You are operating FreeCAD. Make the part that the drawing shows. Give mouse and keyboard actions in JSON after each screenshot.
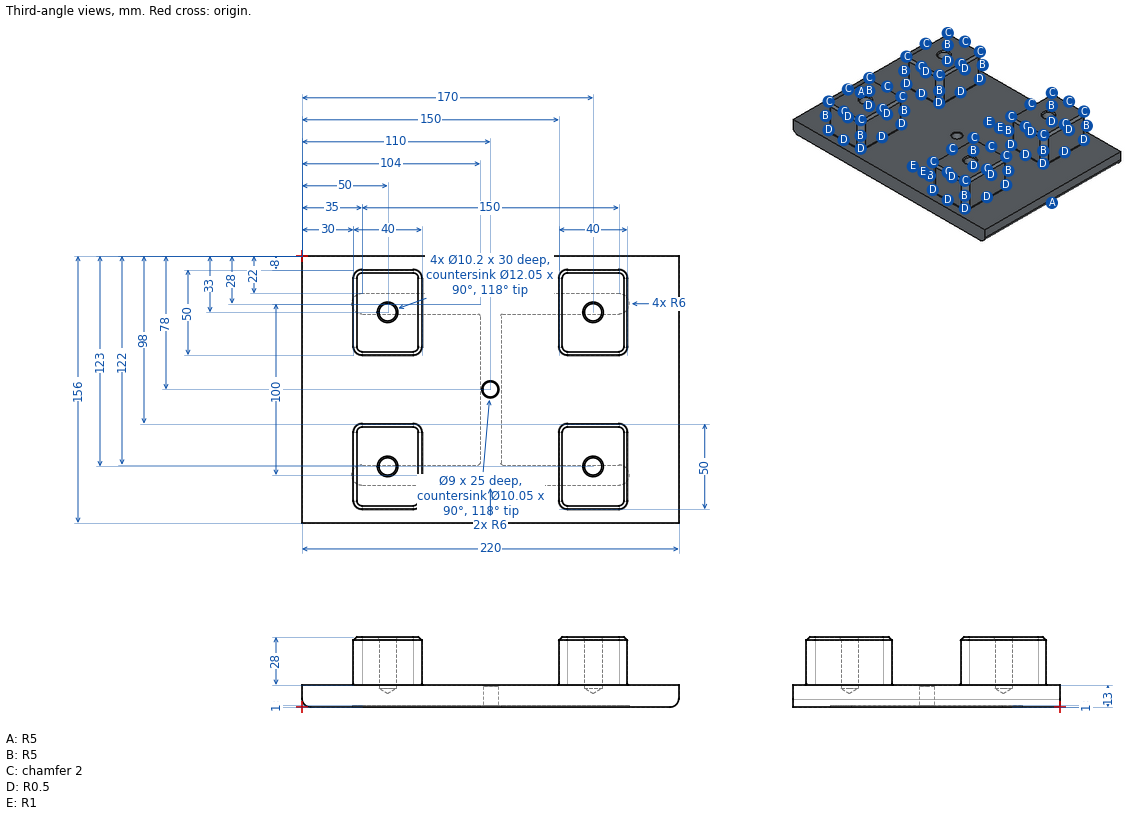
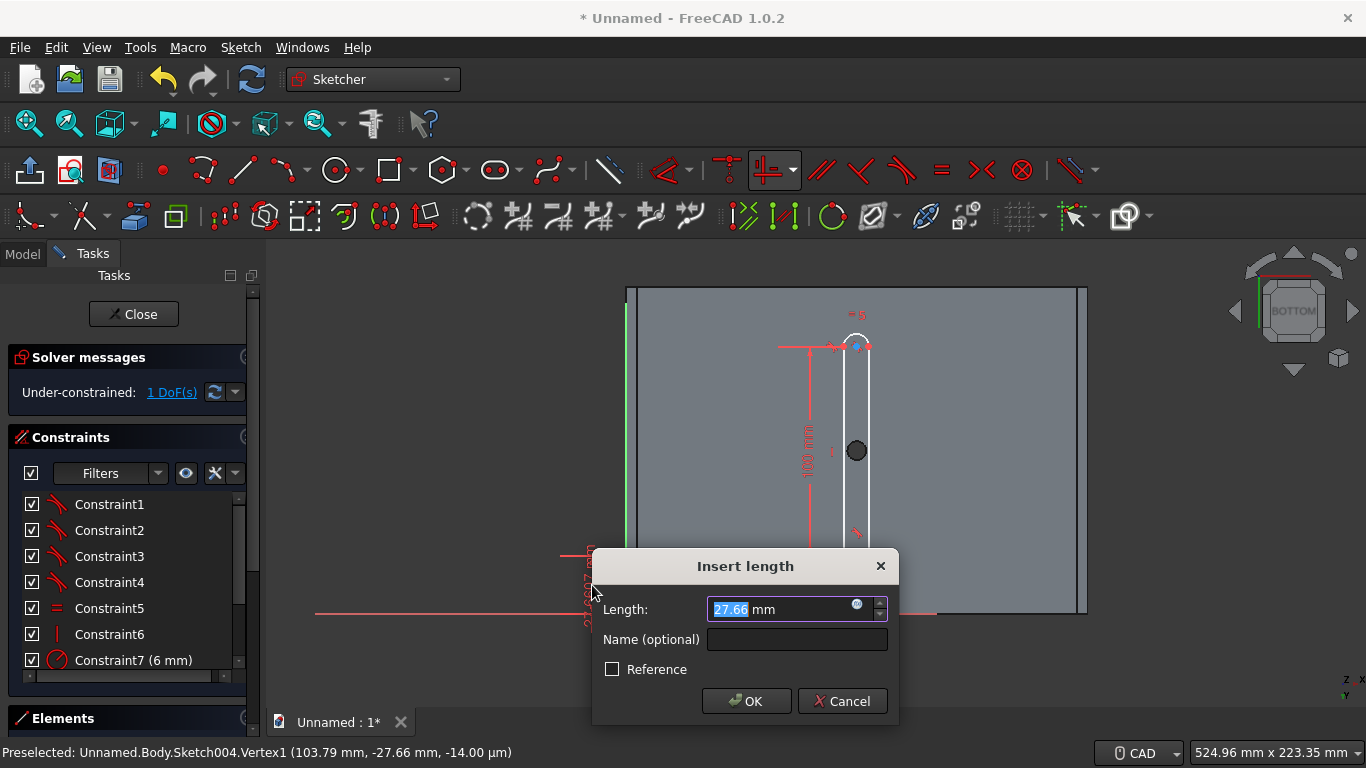
{"action": "type", "text": "28"}
{"action": "key", "text": "Return"}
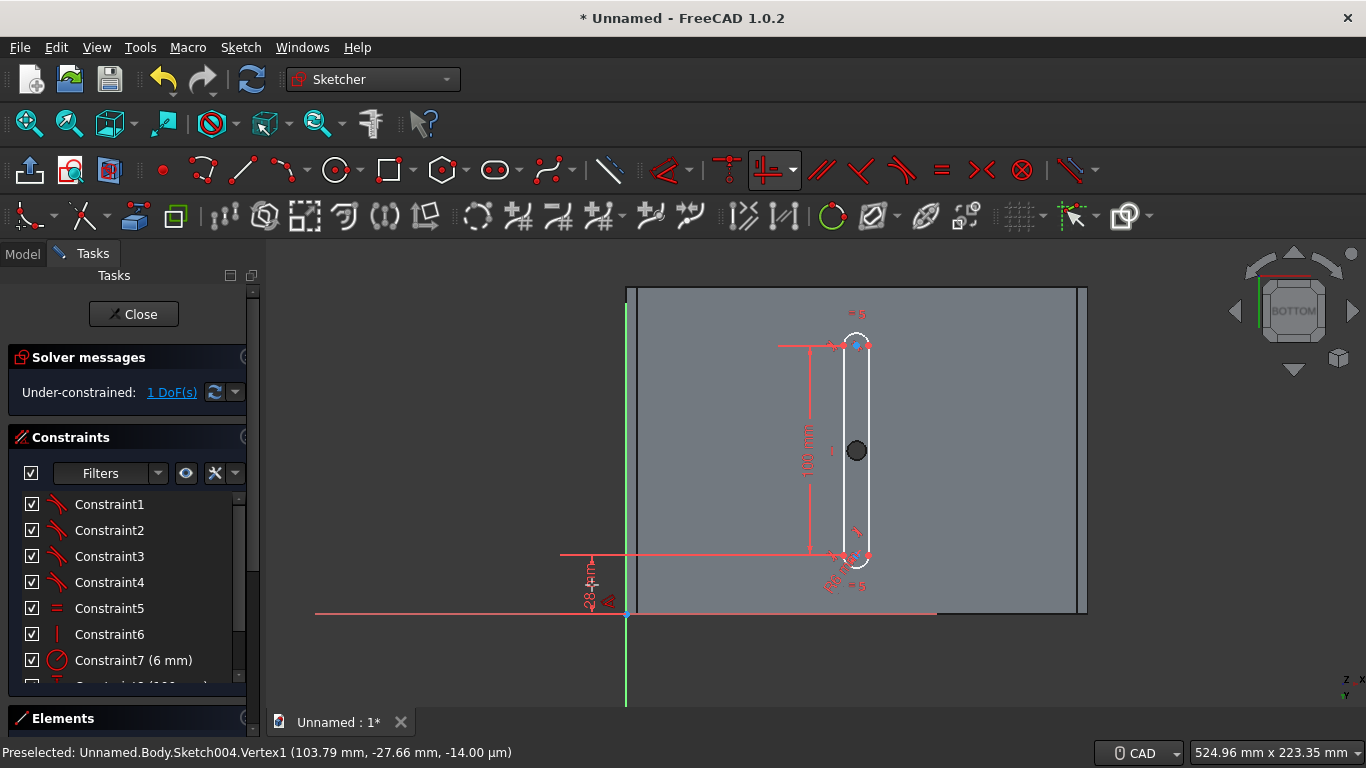
{"action": "left_click", "coordinate": [844, 555]}
{"action": "left_click", "coordinate": [735, 648]}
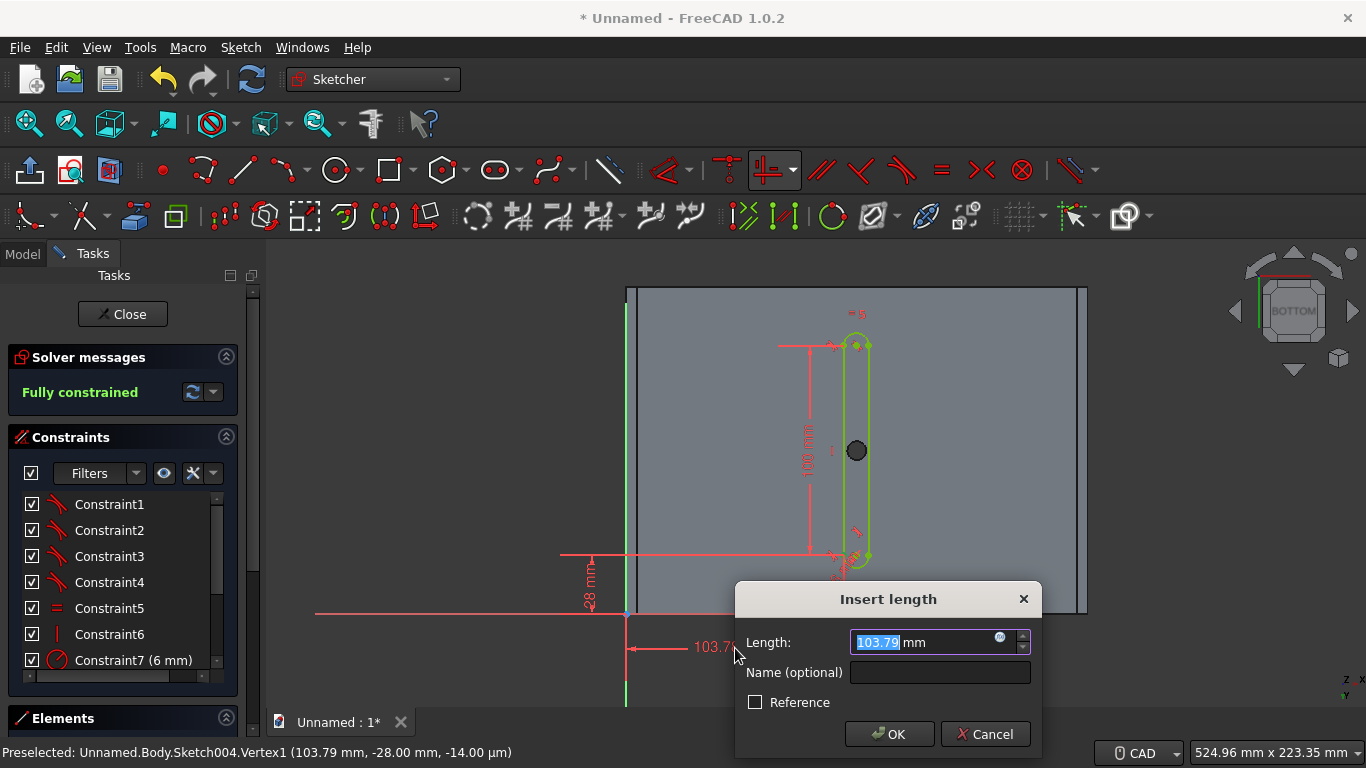
{"action": "type", "text": "104"}
{"action": "key", "text": "Return"}
{"action": "key", "text": "Escape"}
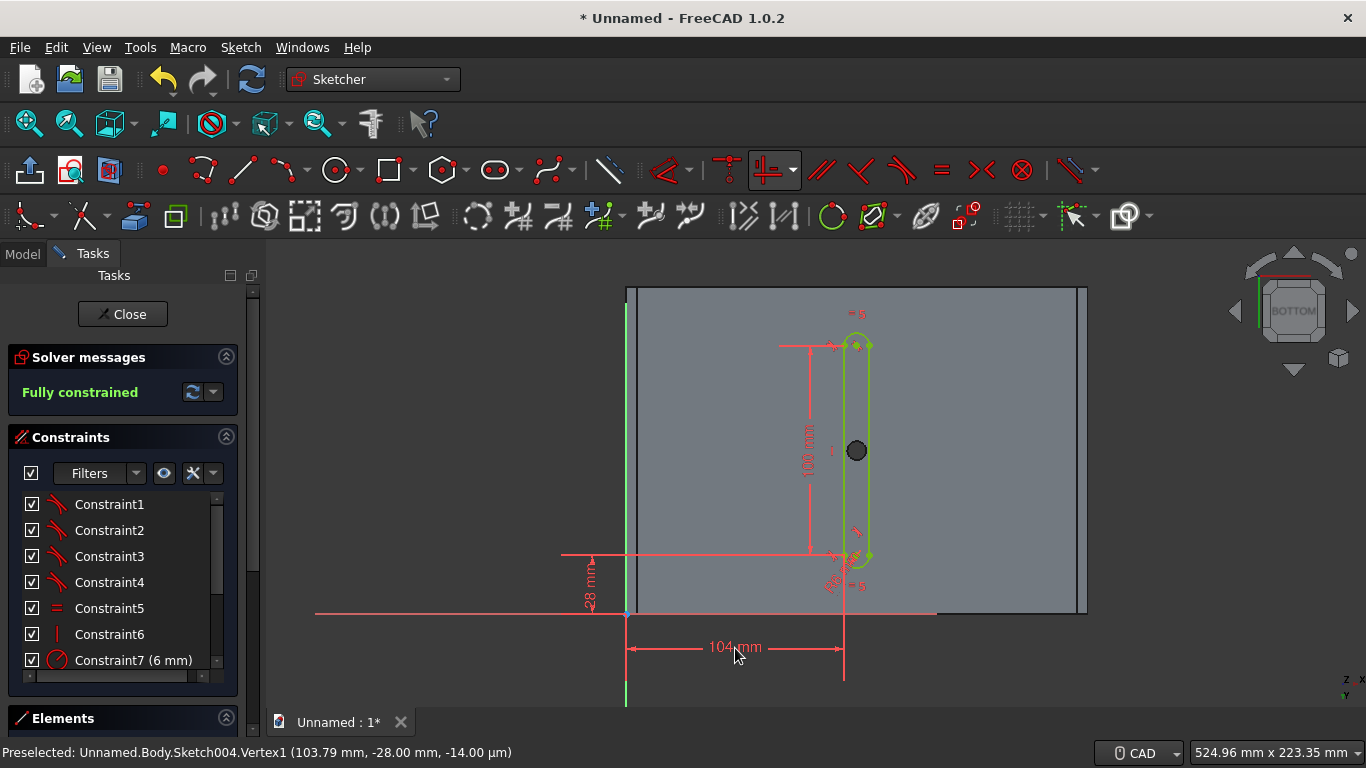
{"action": "left_click", "coordinate": [123, 314]}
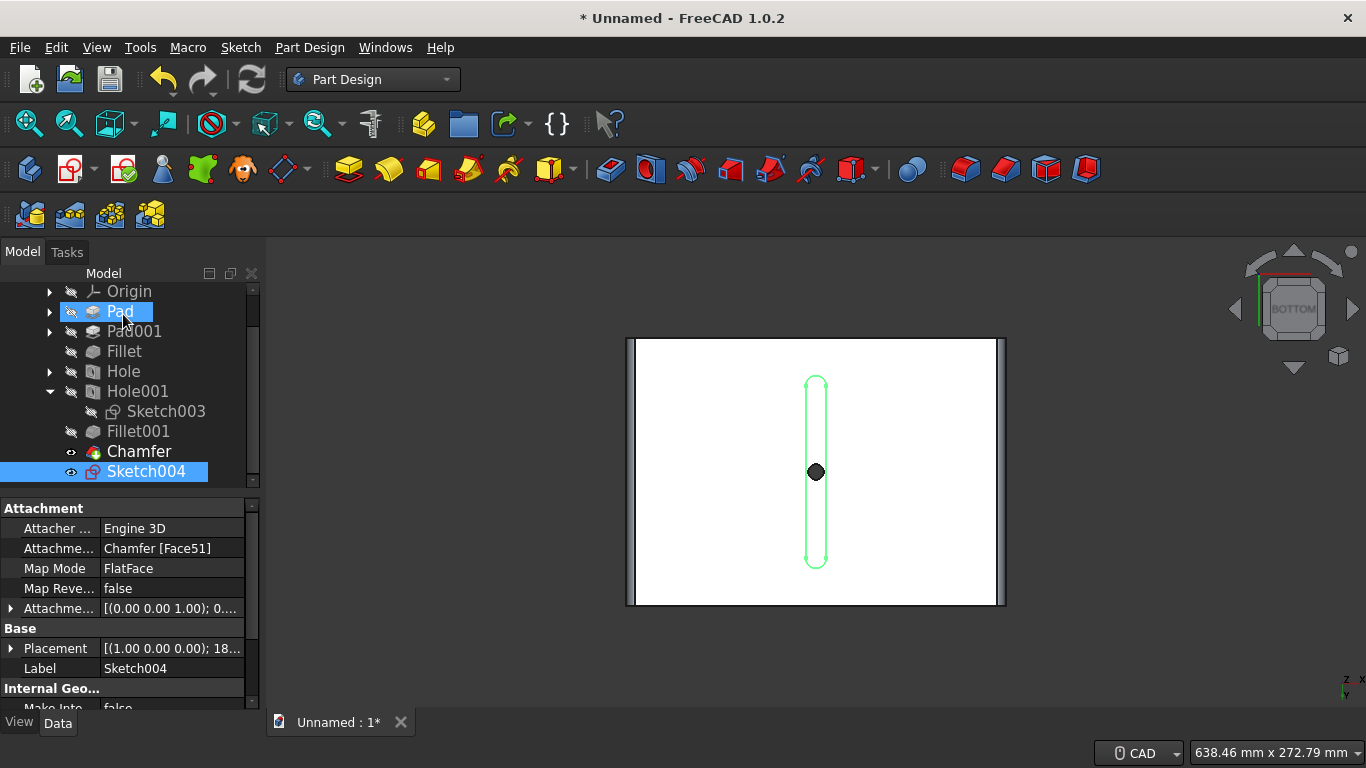
{"action": "left_click", "coordinate": [612, 170]}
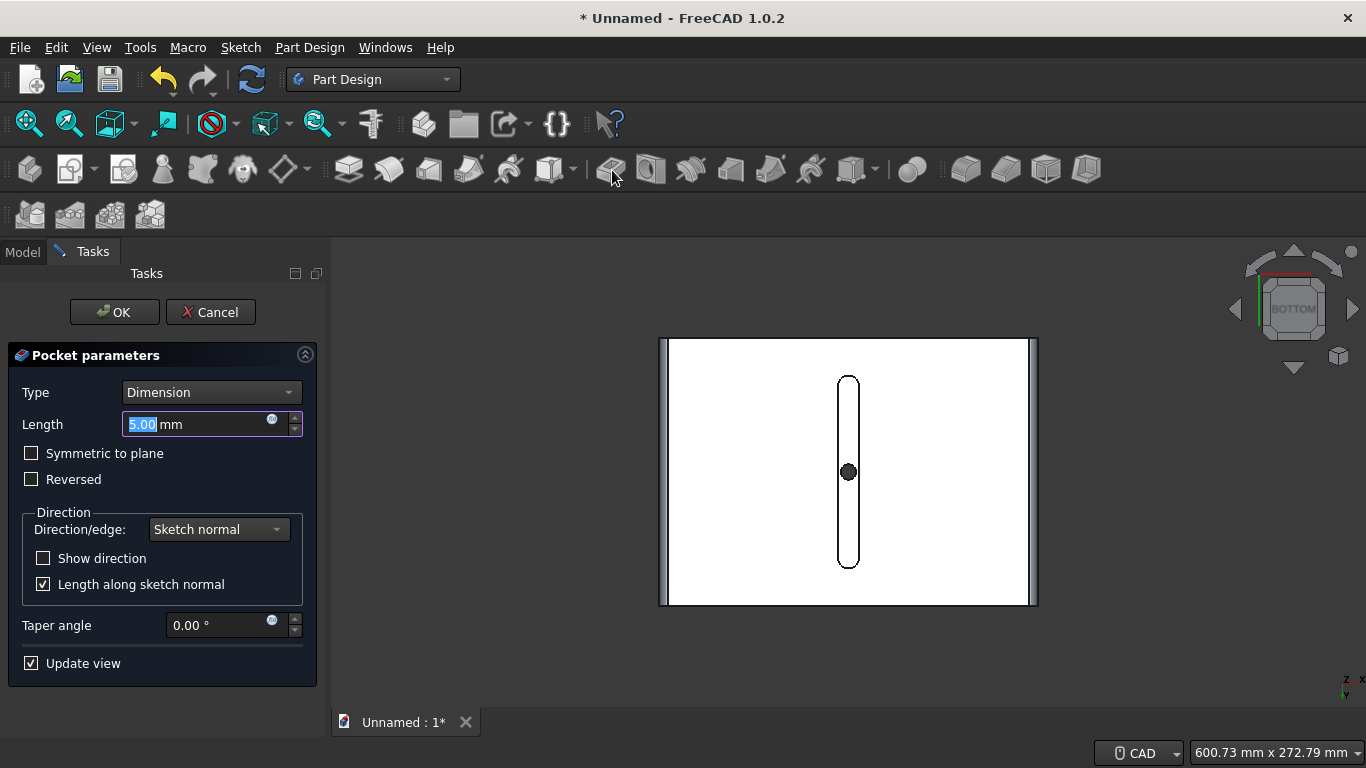
{"action": "type", "text": "1"}
{"action": "key", "text": "Tab"}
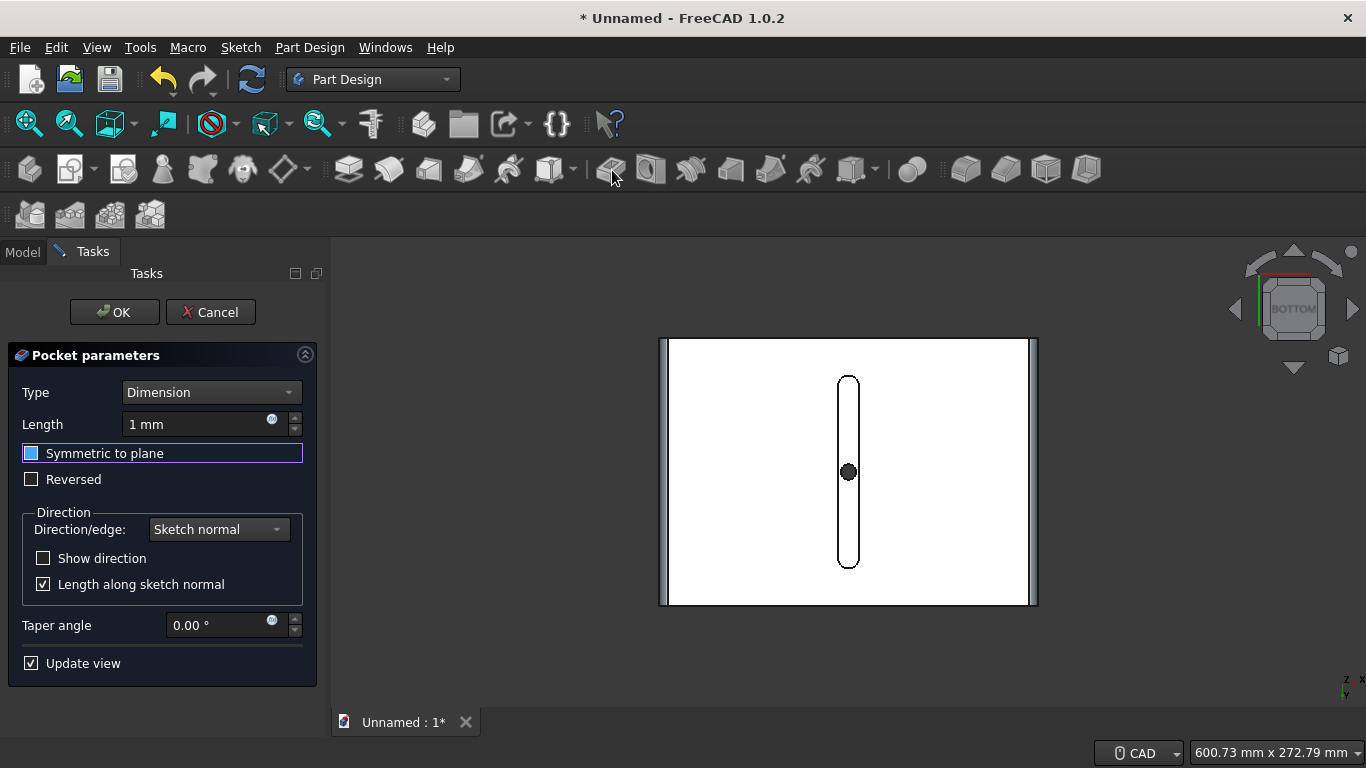
{"action": "left_click", "coordinate": [115, 312]}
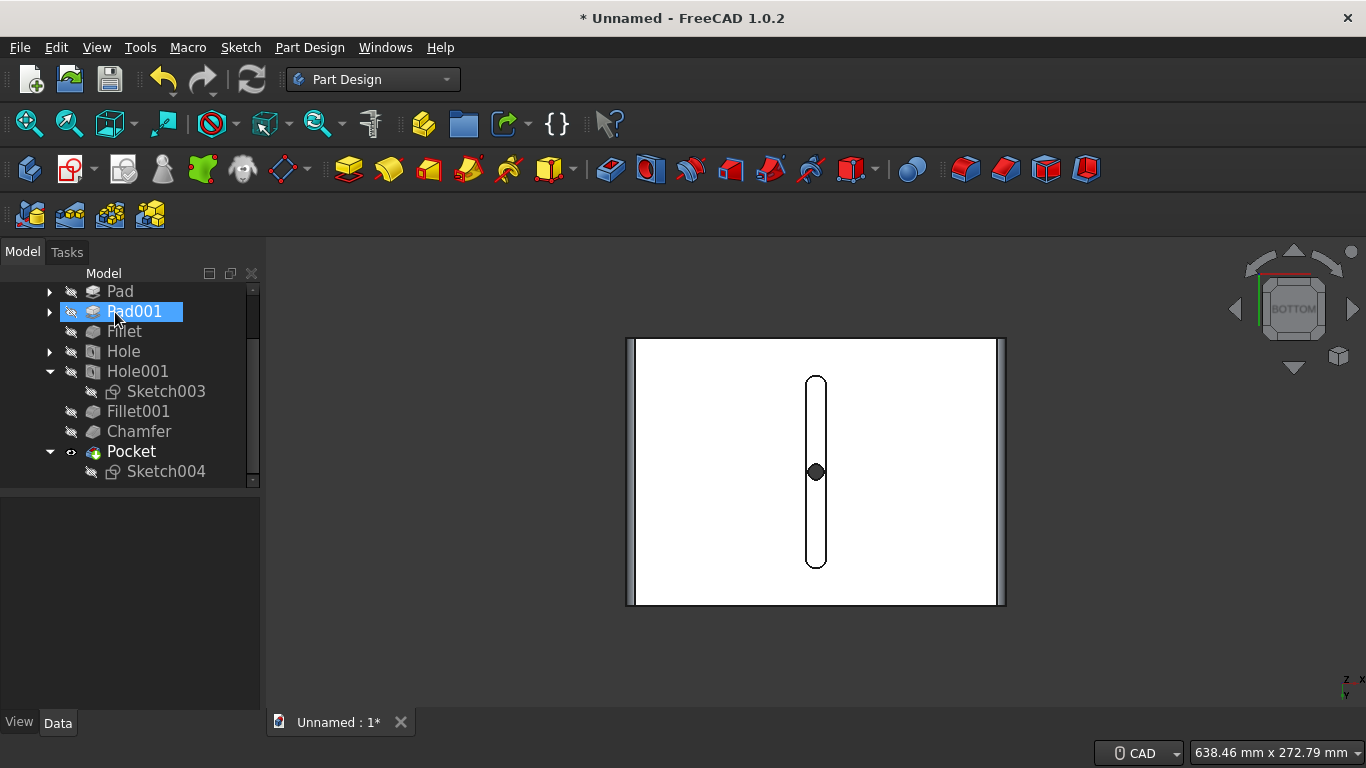
{"action": "left_click", "coordinate": [70, 170]}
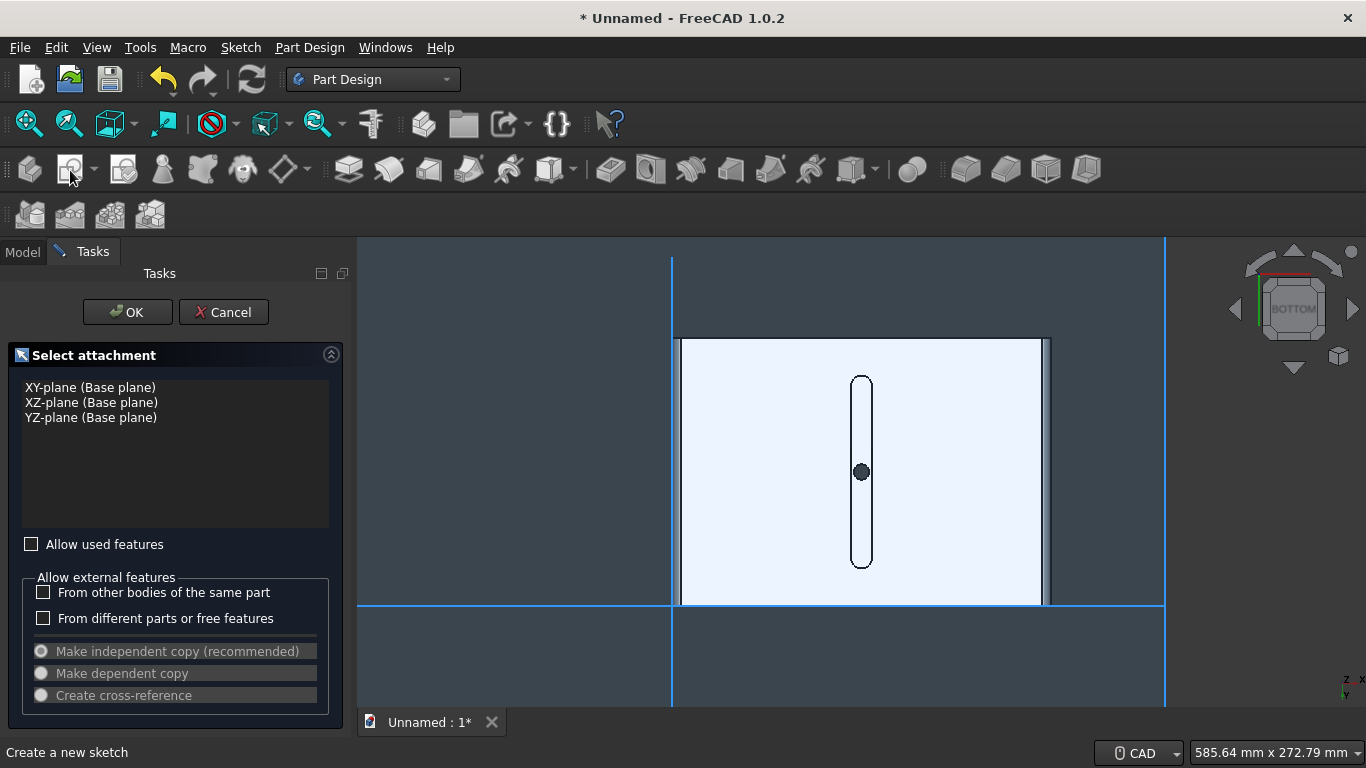
{"action": "left_click", "coordinate": [82, 388]}